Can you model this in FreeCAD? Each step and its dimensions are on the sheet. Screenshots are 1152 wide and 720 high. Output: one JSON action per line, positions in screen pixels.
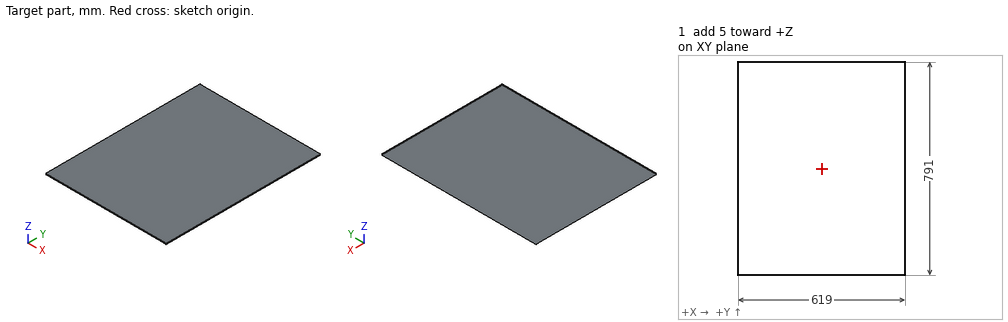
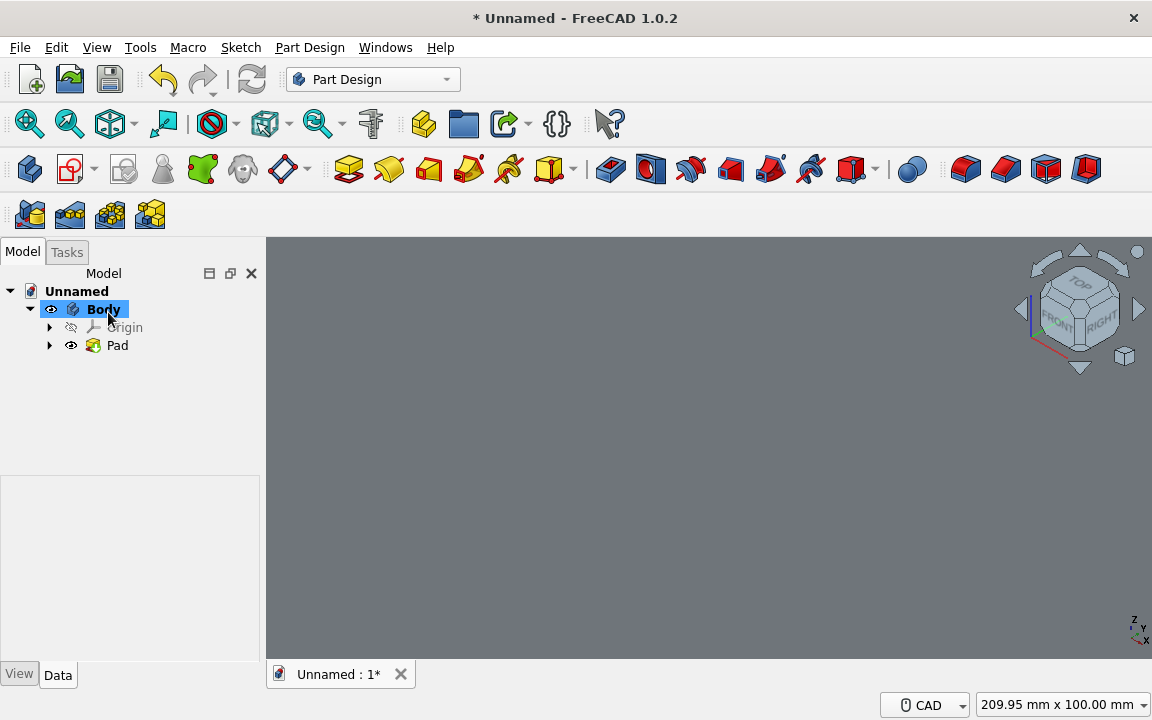
{"action": "left_click", "coordinate": [30, 124]}